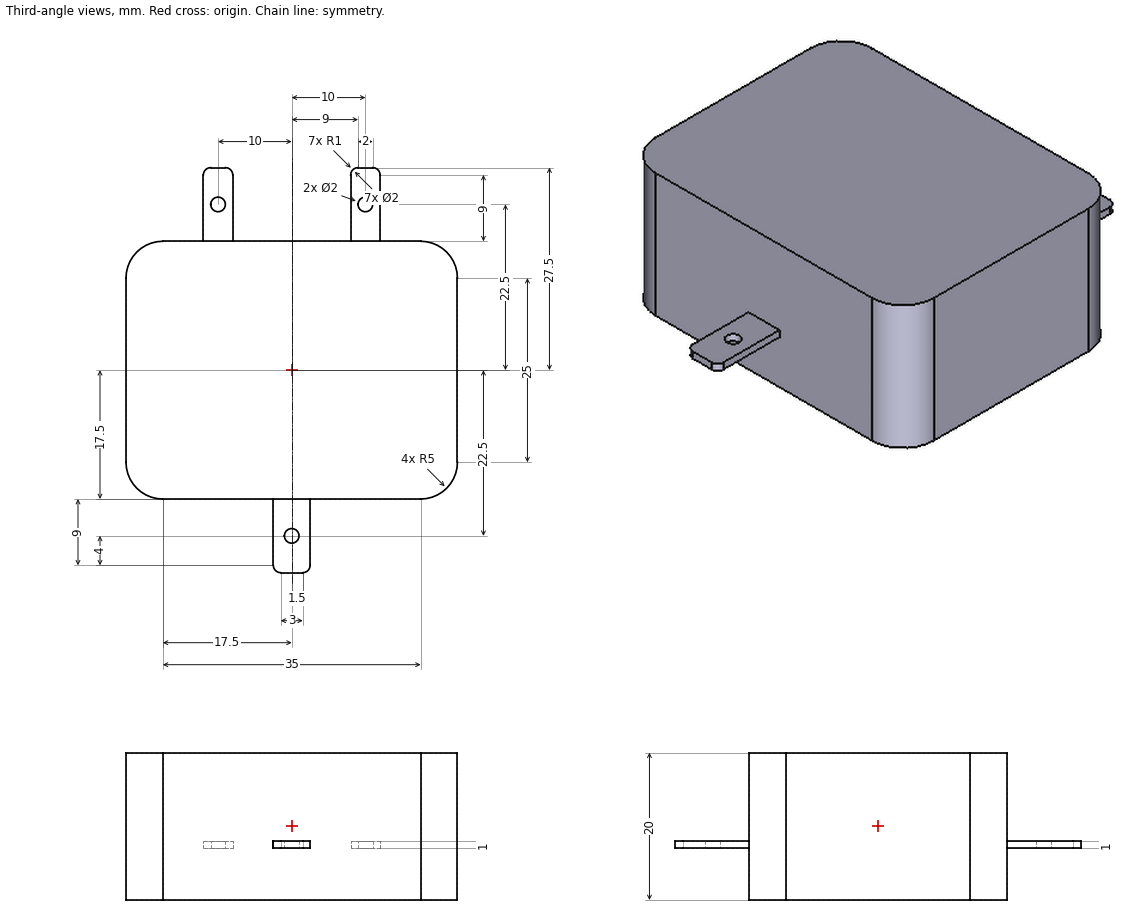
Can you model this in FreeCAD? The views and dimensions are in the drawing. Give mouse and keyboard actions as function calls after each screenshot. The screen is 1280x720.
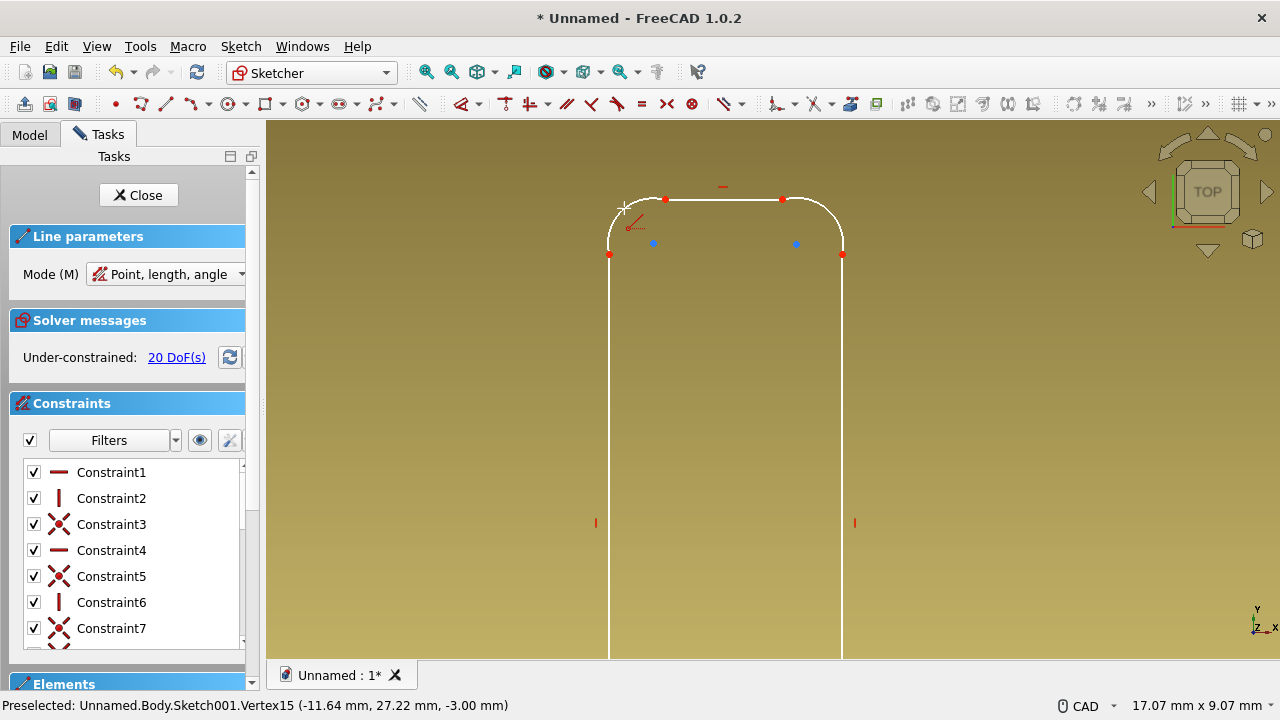
scroll(628, 211, down, 11)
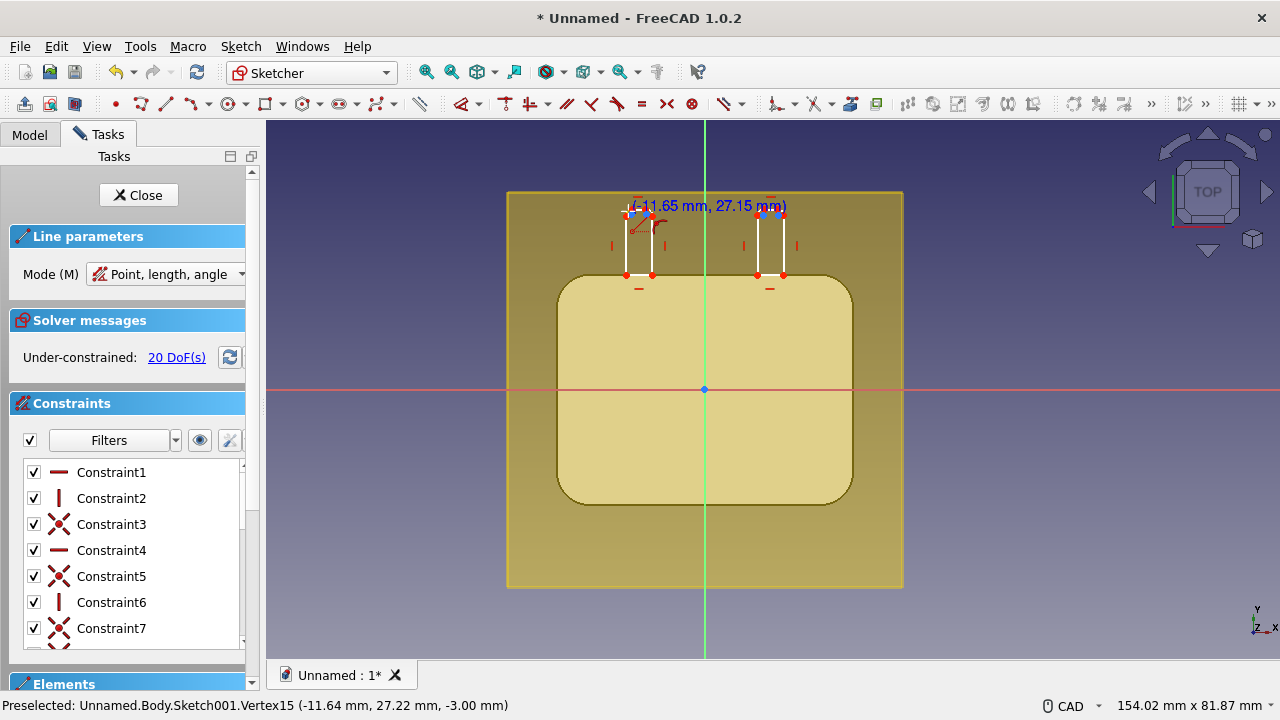
scroll(715, 571, up, 3)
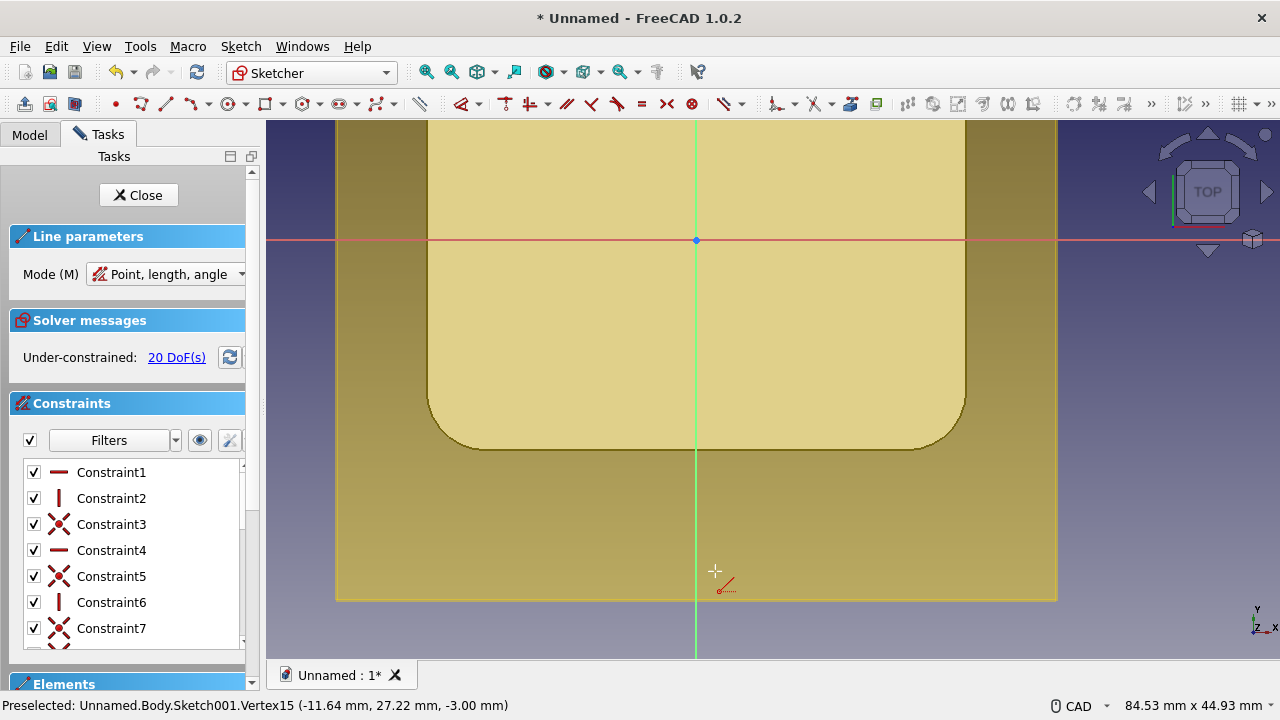
click(714, 570)
click(678, 570)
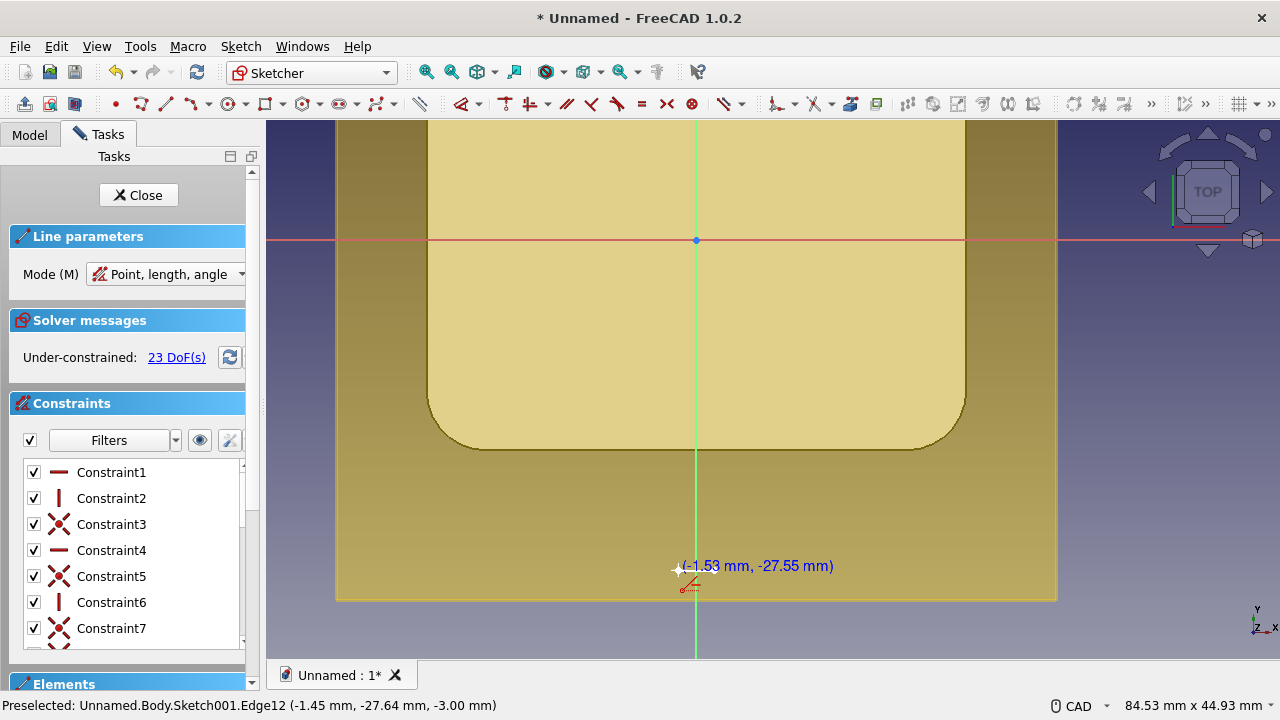
click(141, 104)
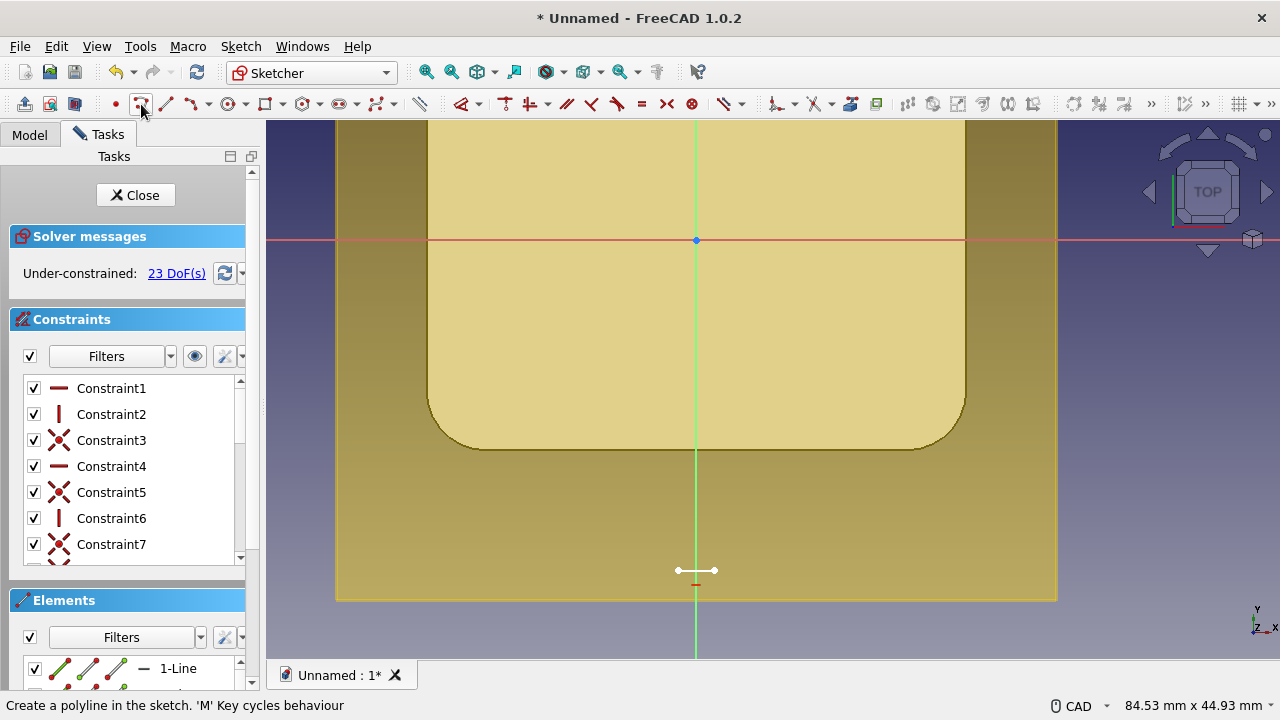
click(666, 558)
click(666, 450)
click(726, 450)
click(726, 558)
right_click(726, 558)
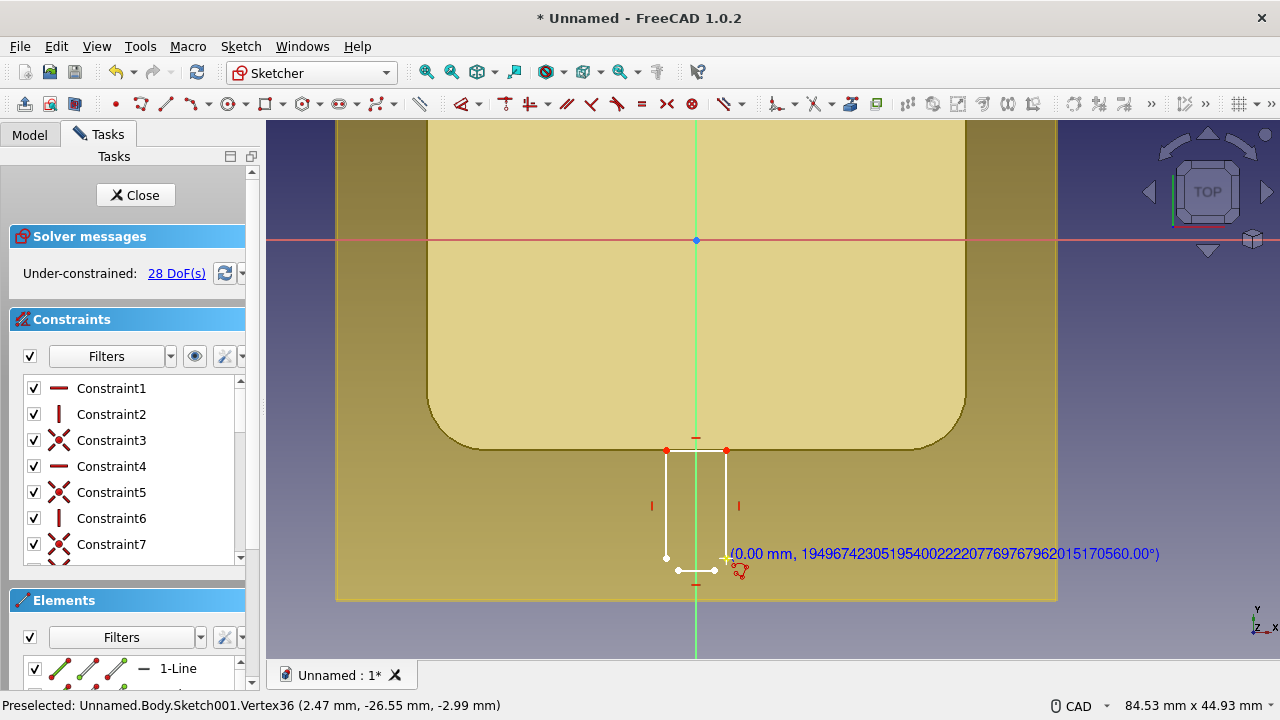
click(190, 104)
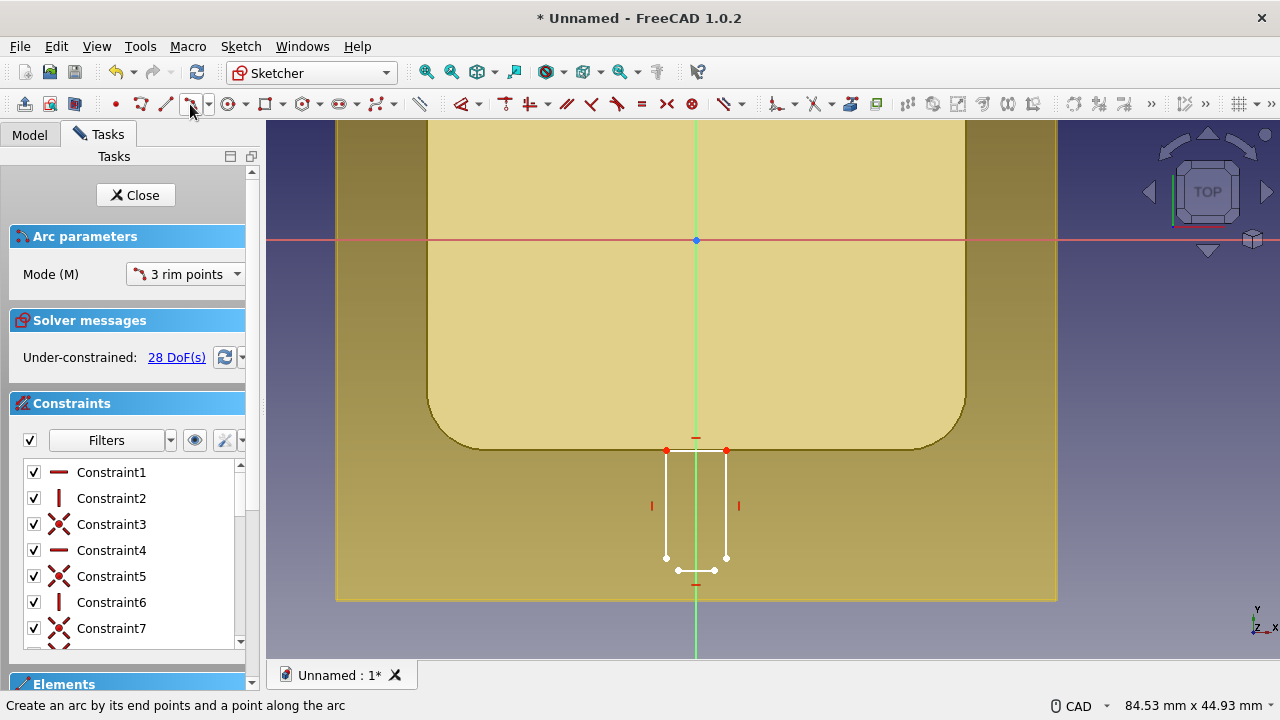
click(678, 571)
click(666, 559)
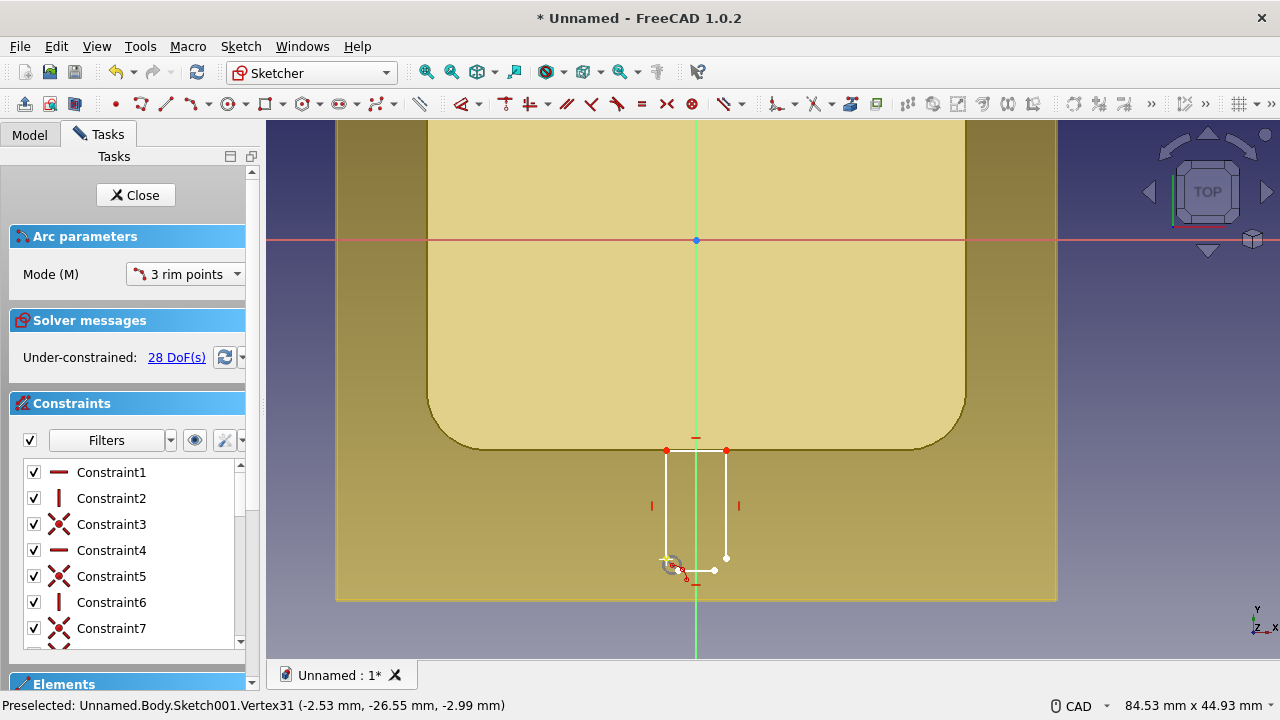
scroll(670, 567, up, 8)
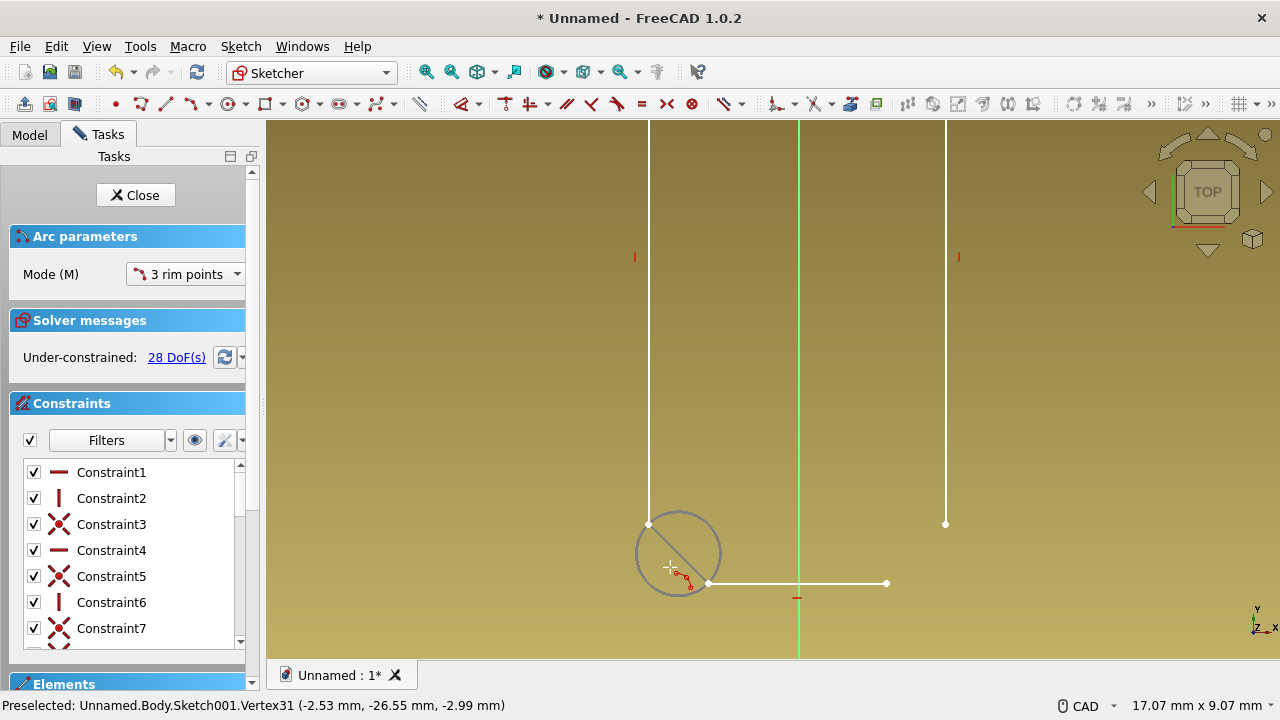
click(668, 563)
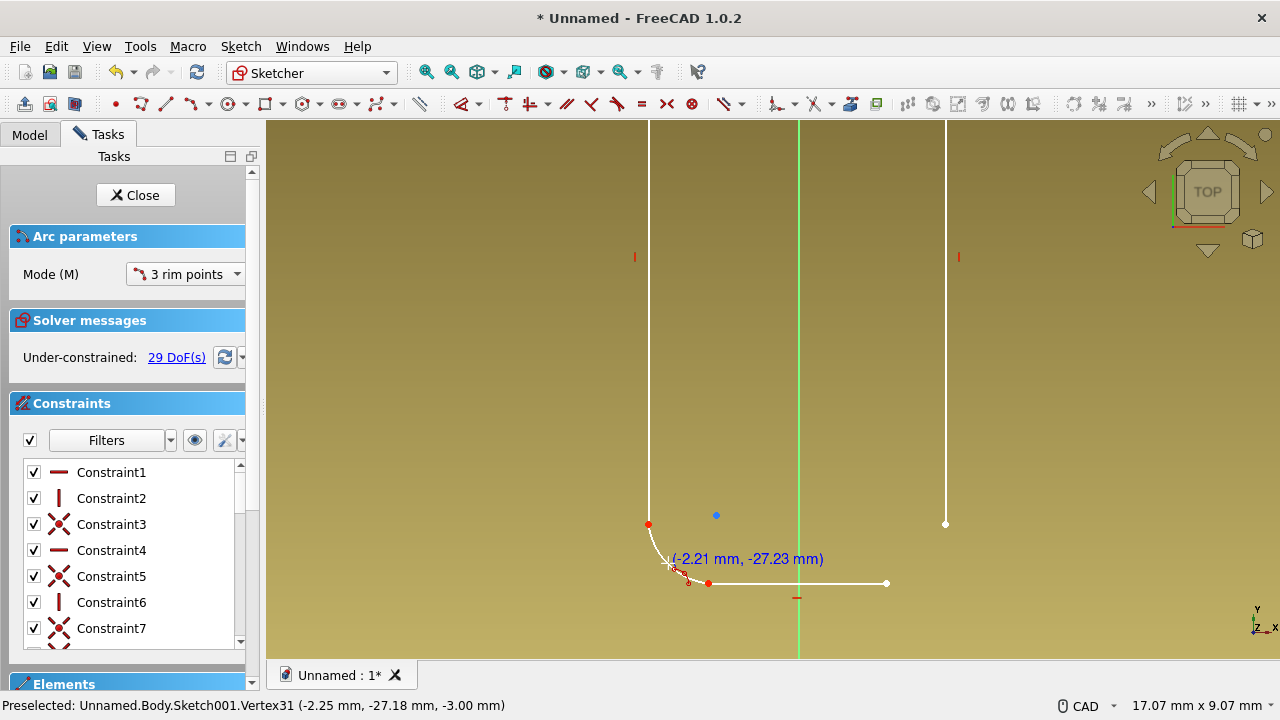
scroll(693, 569, down, 11)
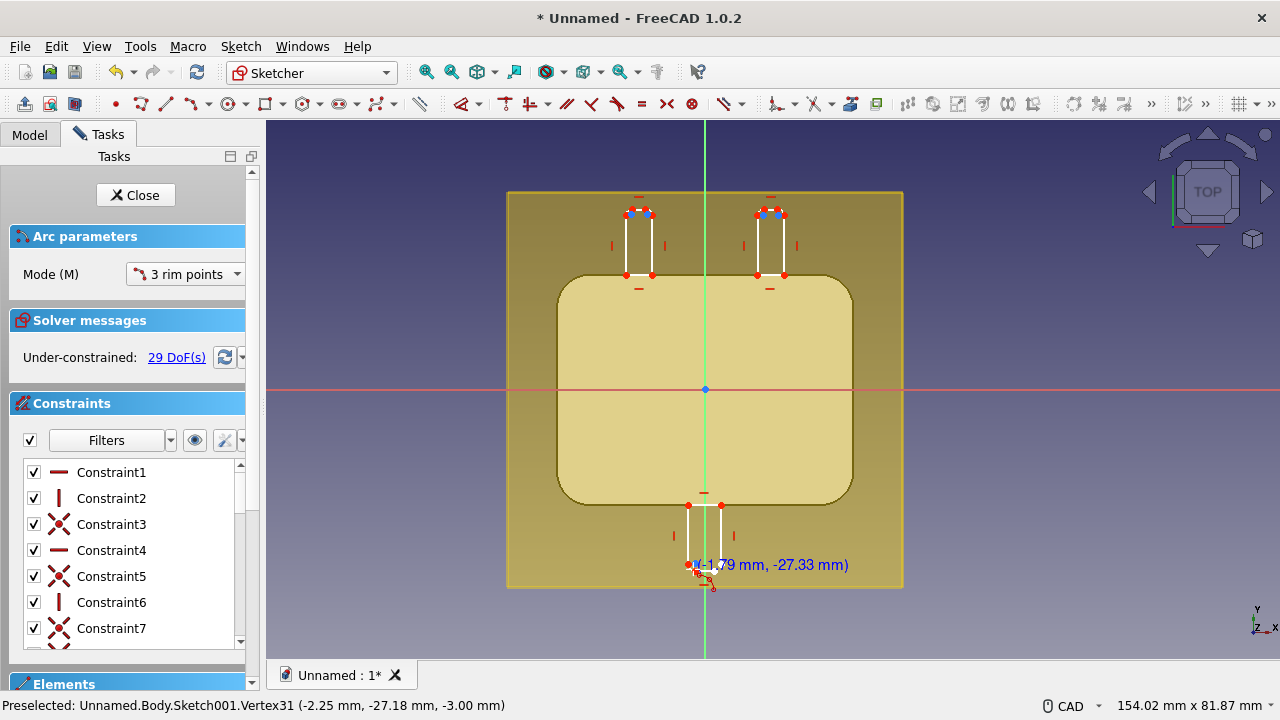
scroll(722, 564, up, 3)